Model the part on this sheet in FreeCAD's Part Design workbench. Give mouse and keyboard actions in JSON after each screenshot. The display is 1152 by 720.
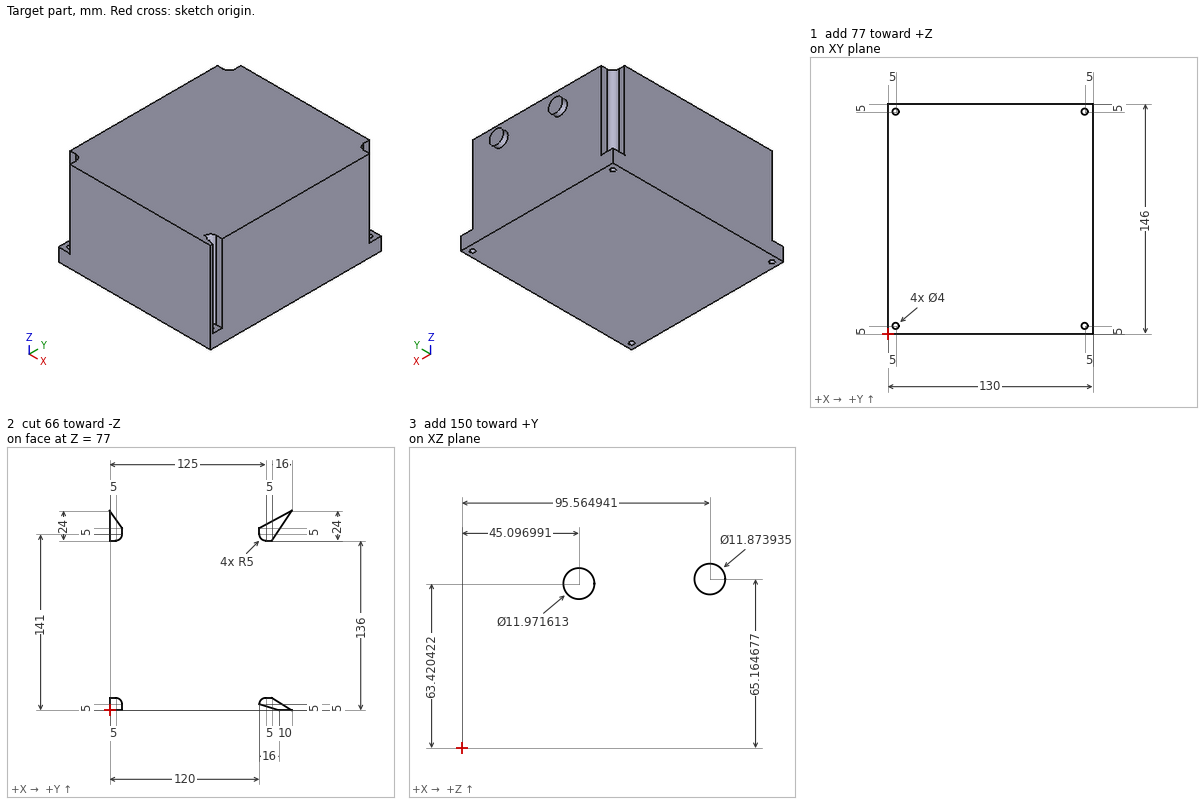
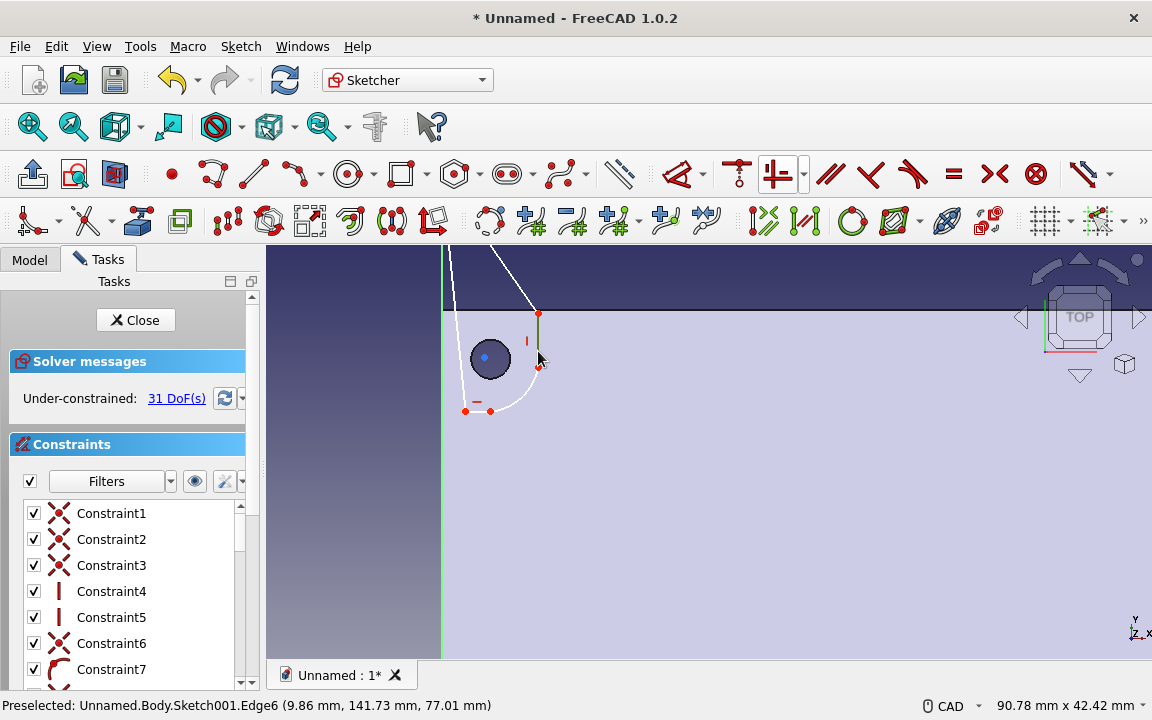
{"action": "left_click", "coordinate": [510, 406]}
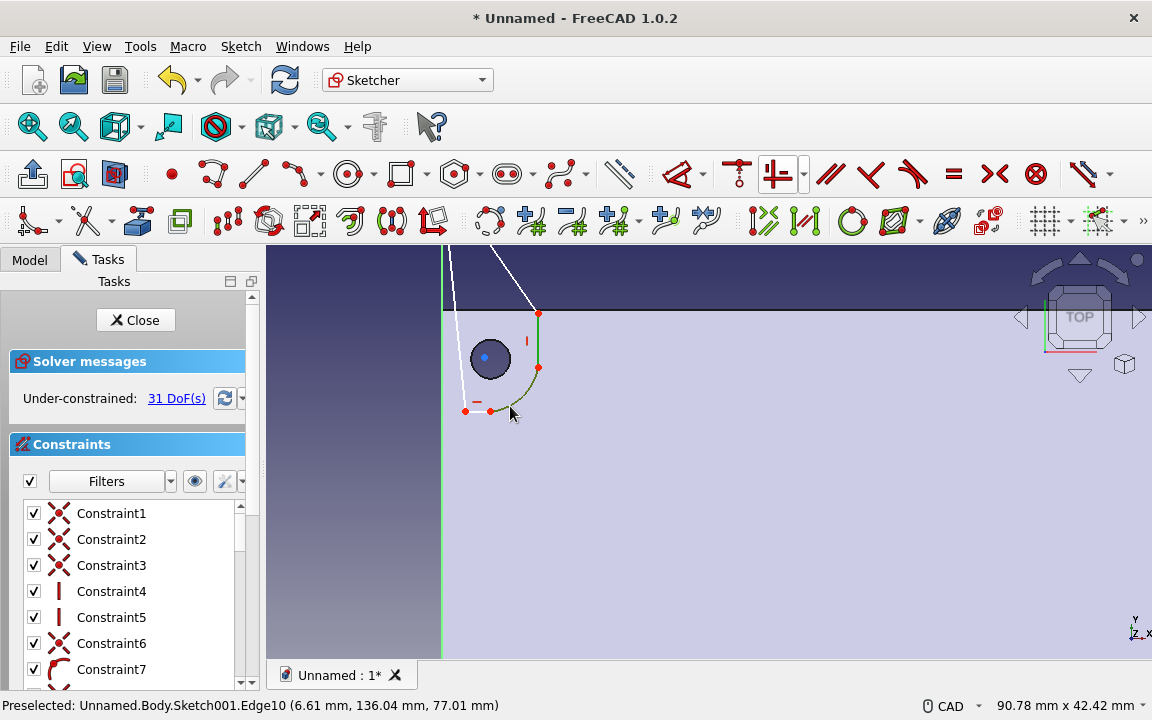
{"action": "left_click", "coordinate": [913, 174]}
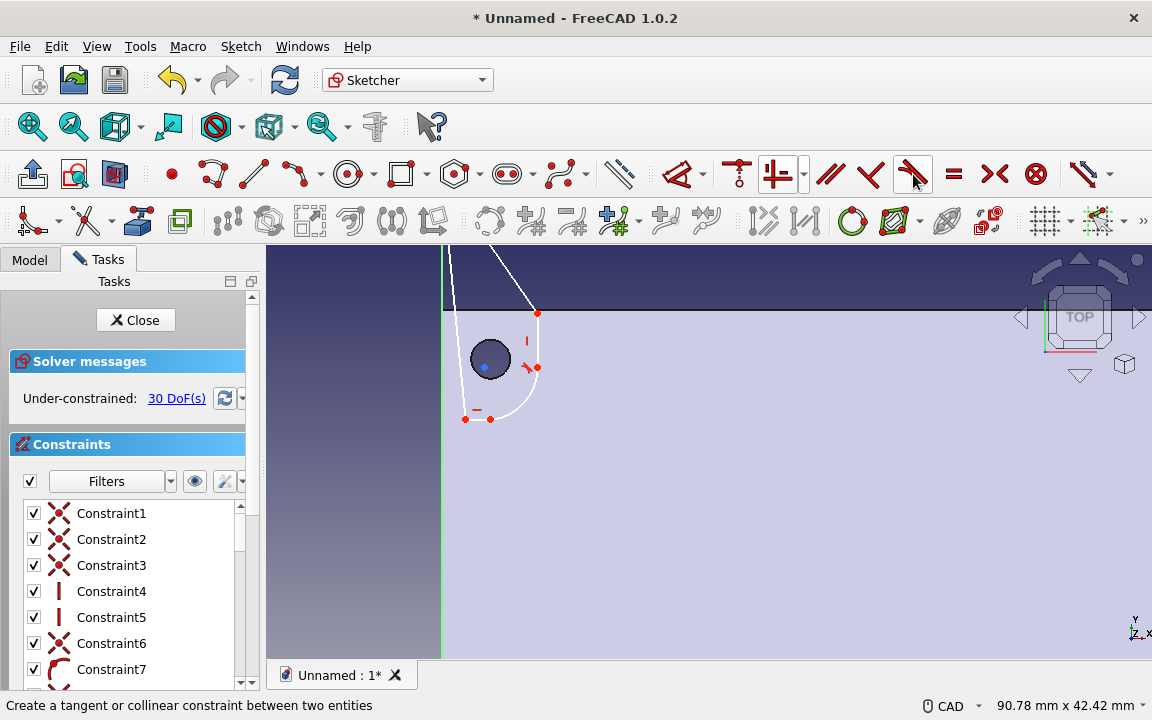
{"action": "scroll", "coordinate": [475, 420], "scroll_direction": "up", "scroll_amount": 2}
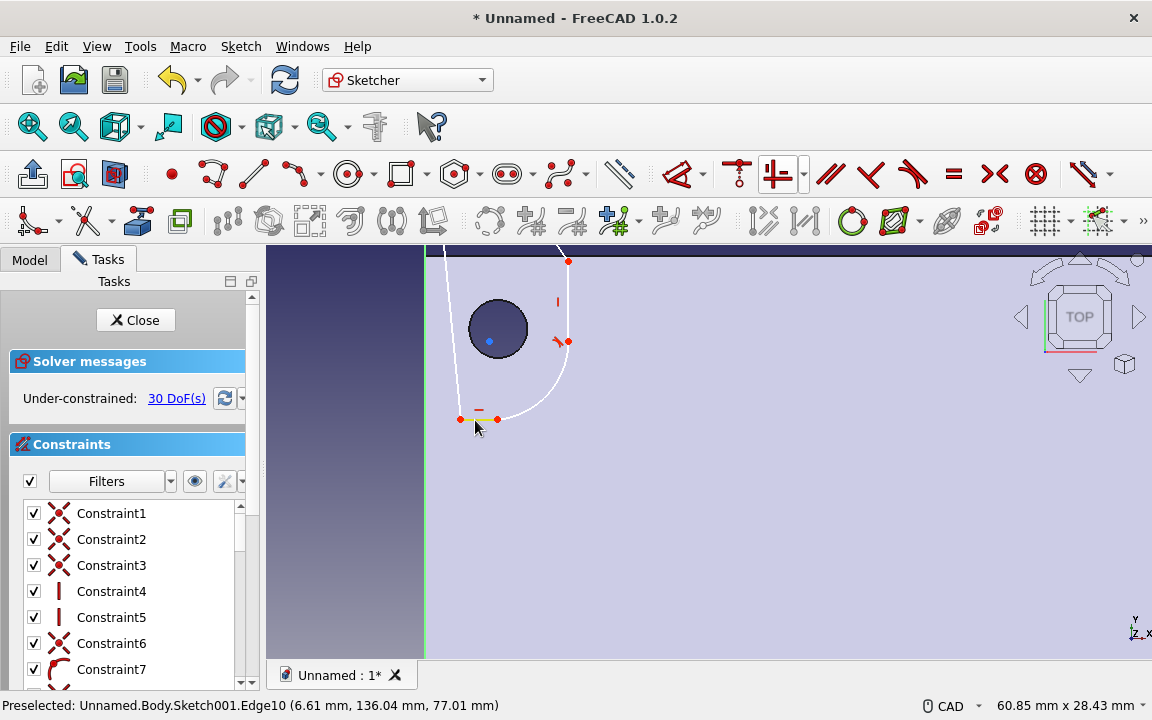
{"action": "left_click", "coordinate": [476, 420]}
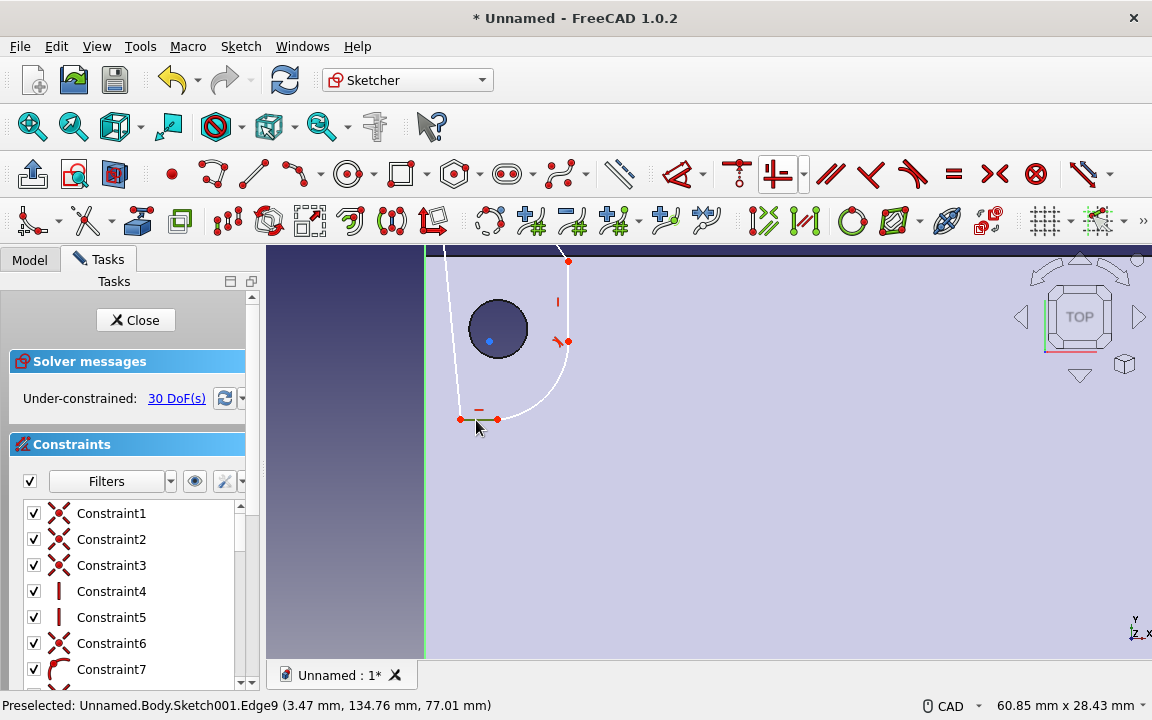
{"action": "left_click", "coordinate": [530, 409]}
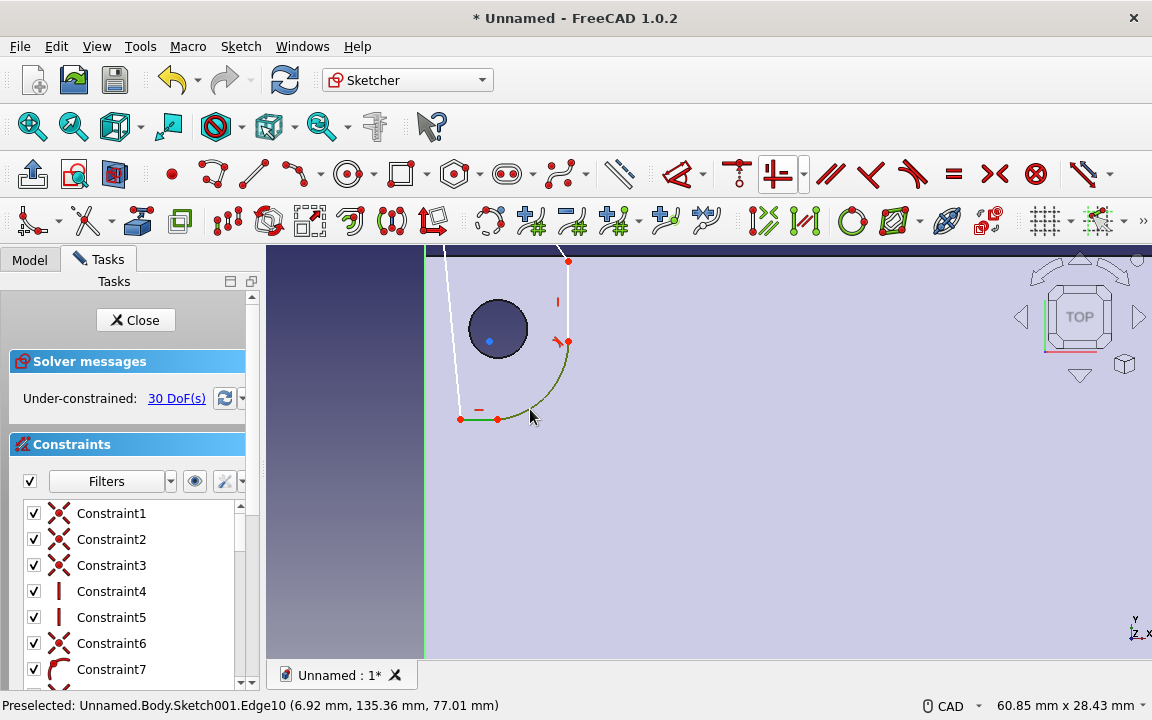
{"action": "left_click", "coordinate": [913, 174]}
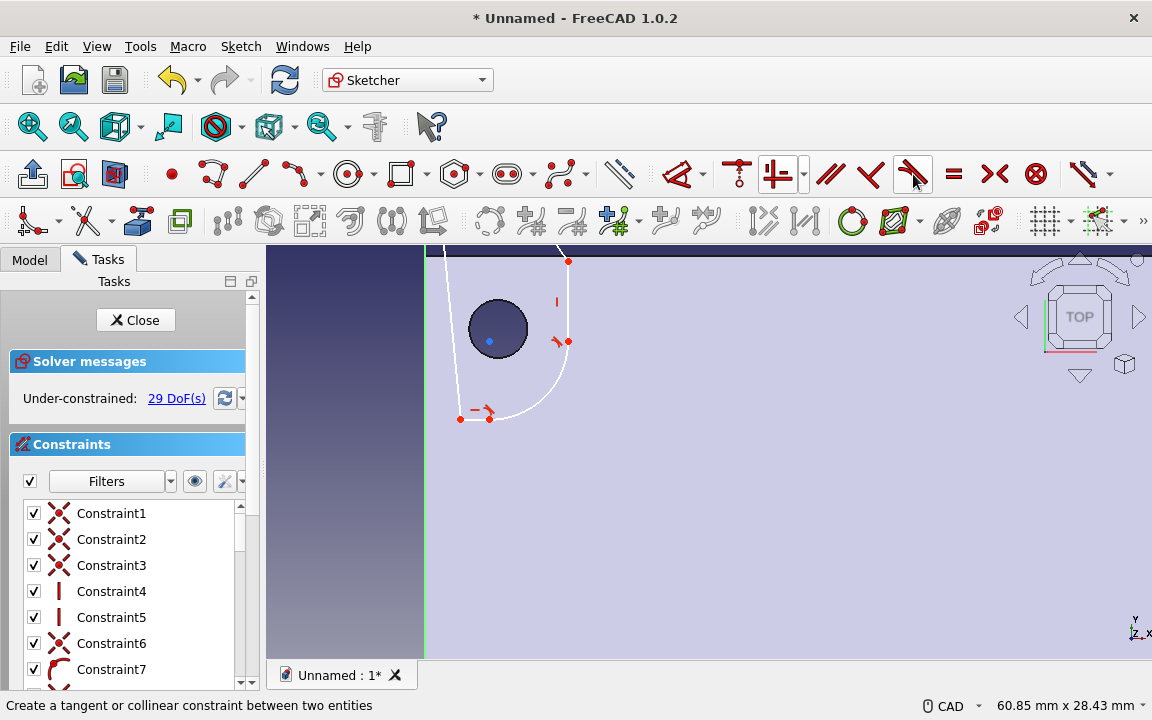
{"action": "scroll", "coordinate": [535, 357], "scroll_direction": "down", "scroll_amount": 11}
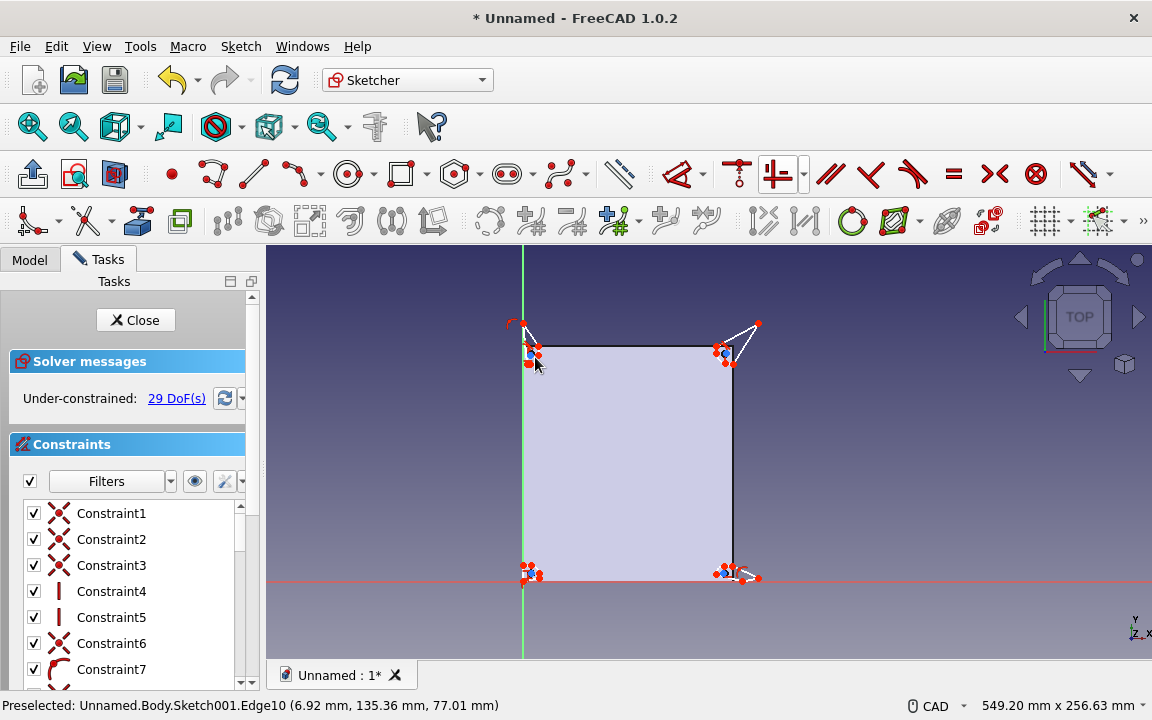
{"action": "scroll", "coordinate": [529, 566], "scroll_direction": "up", "scroll_amount": 9}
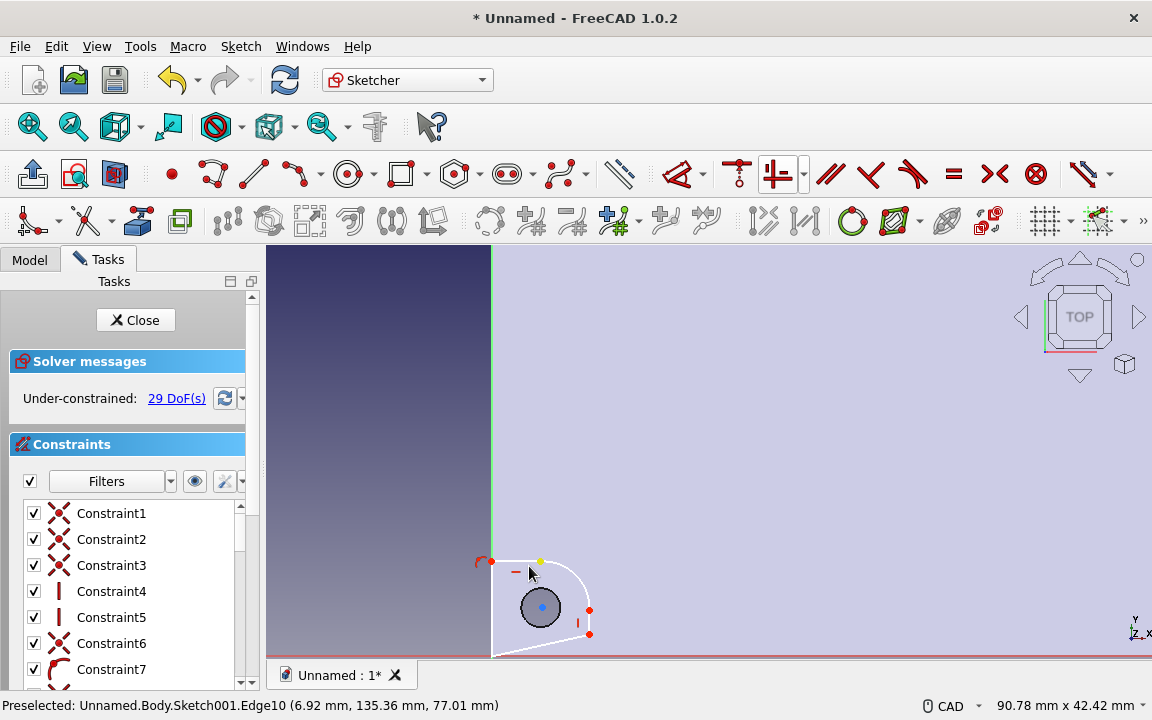
{"action": "left_click", "coordinate": [526, 561]}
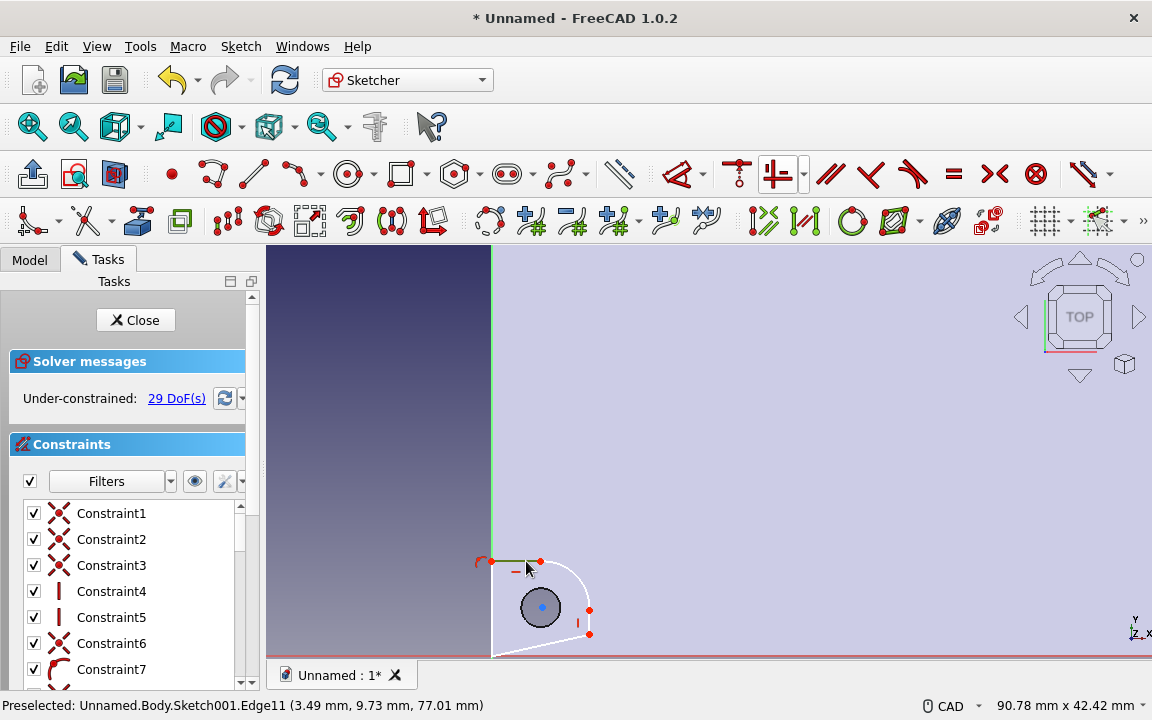
{"action": "left_click", "coordinate": [585, 588]}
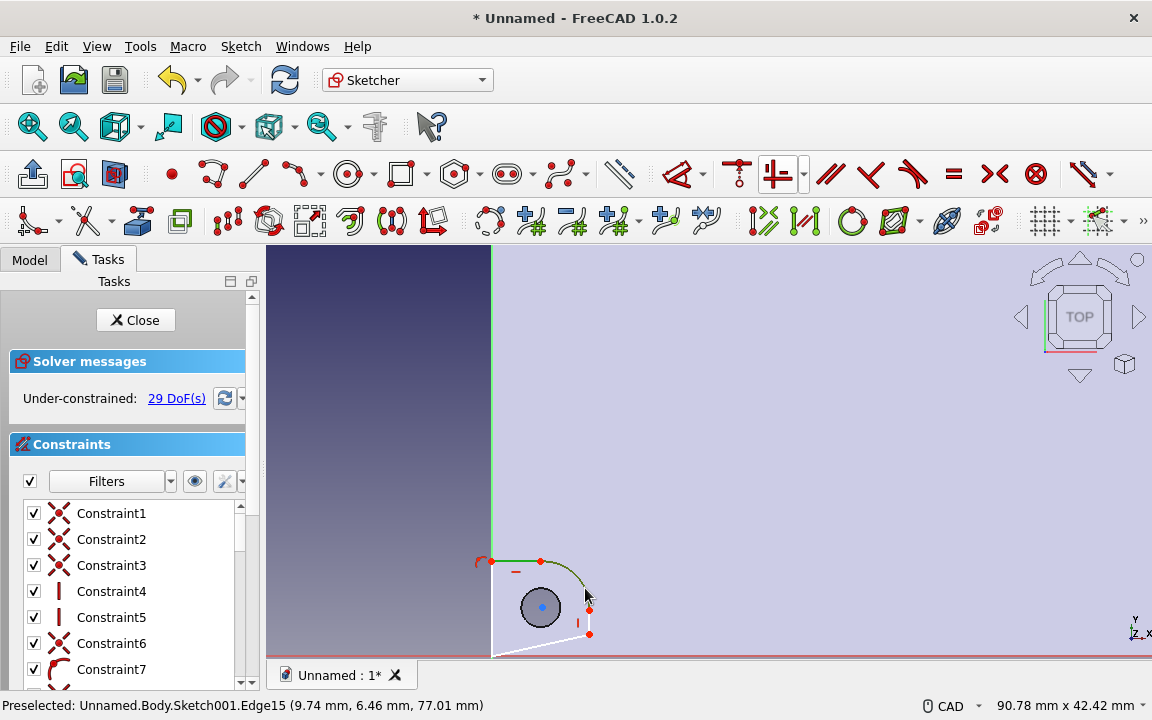
{"action": "left_click", "coordinate": [913, 174]}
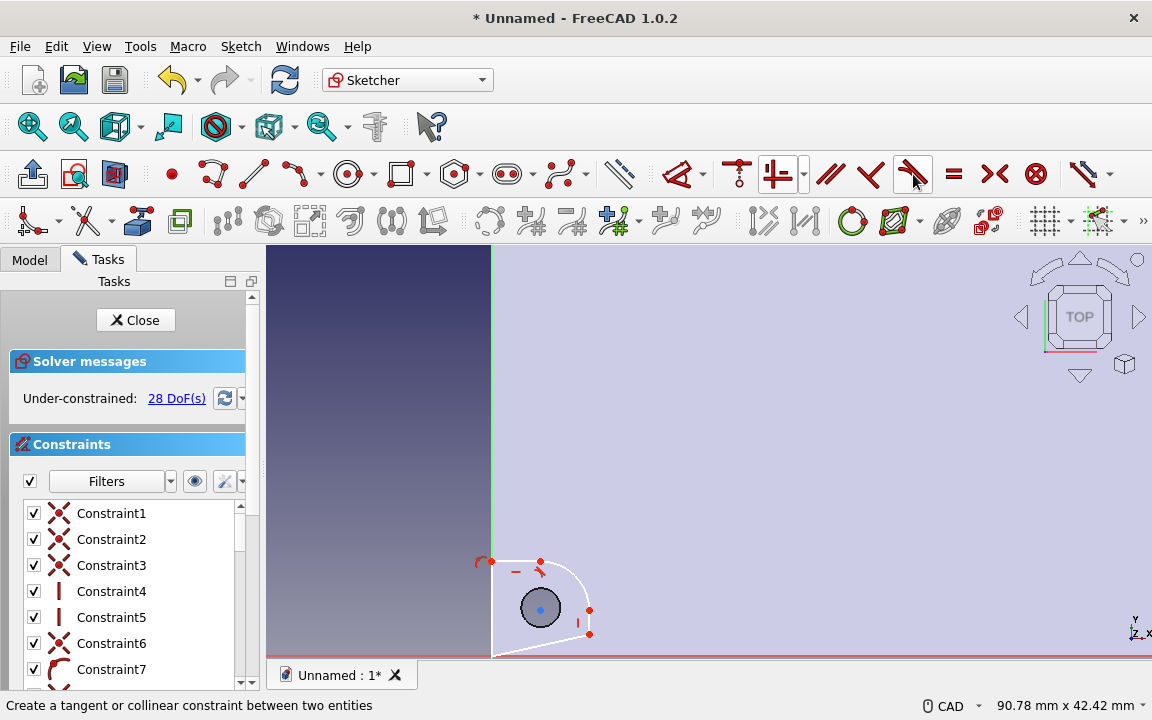
{"action": "scroll", "coordinate": [589, 625], "scroll_direction": "up", "scroll_amount": 2}